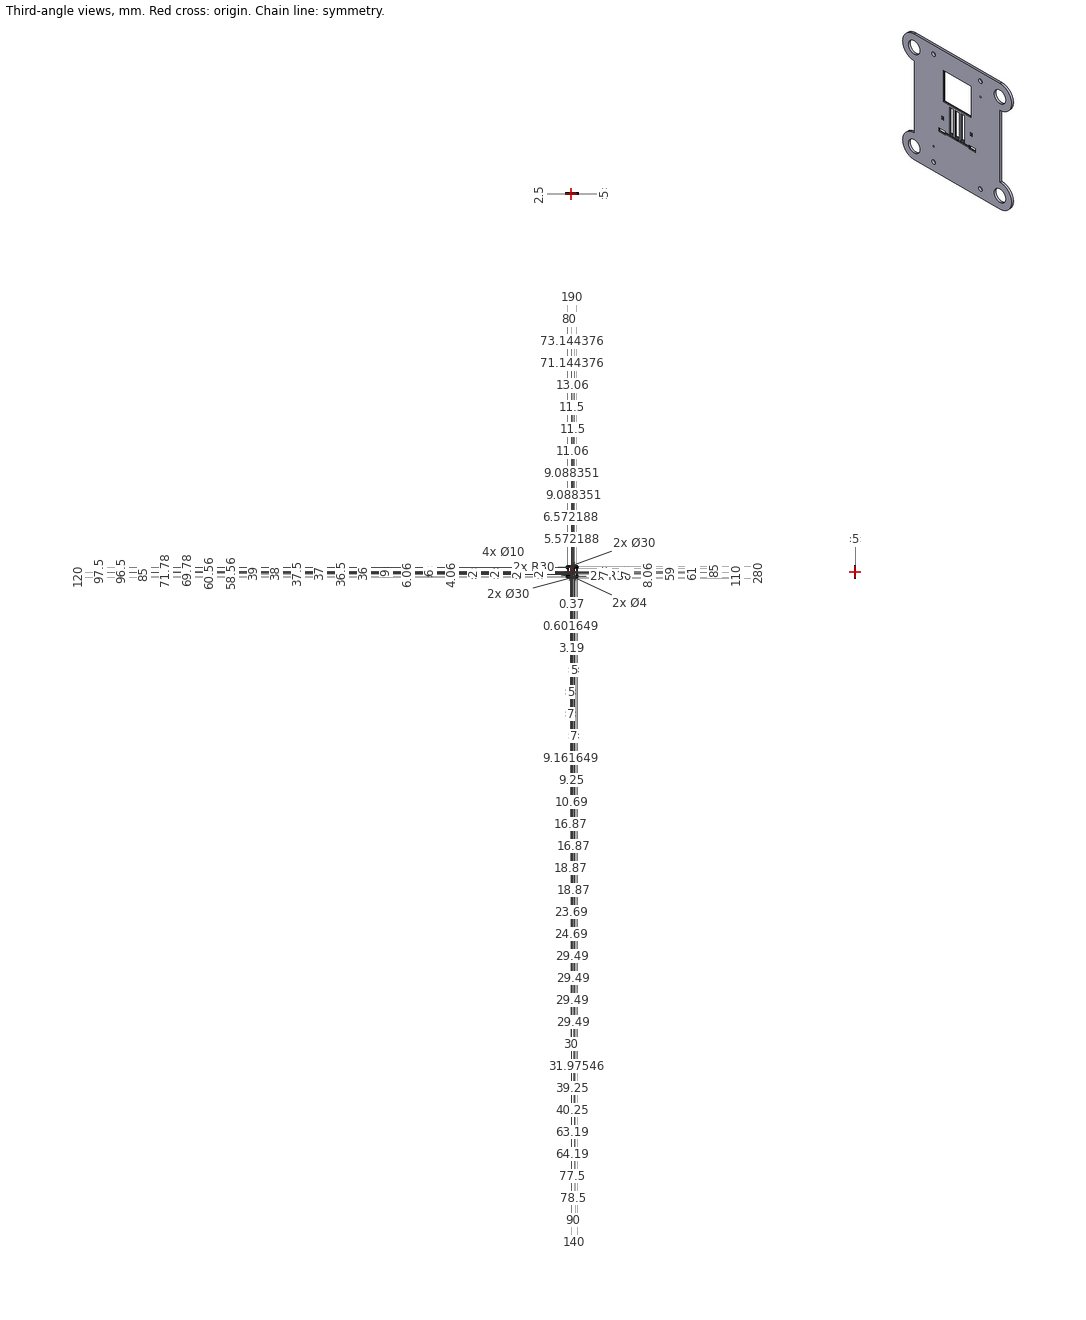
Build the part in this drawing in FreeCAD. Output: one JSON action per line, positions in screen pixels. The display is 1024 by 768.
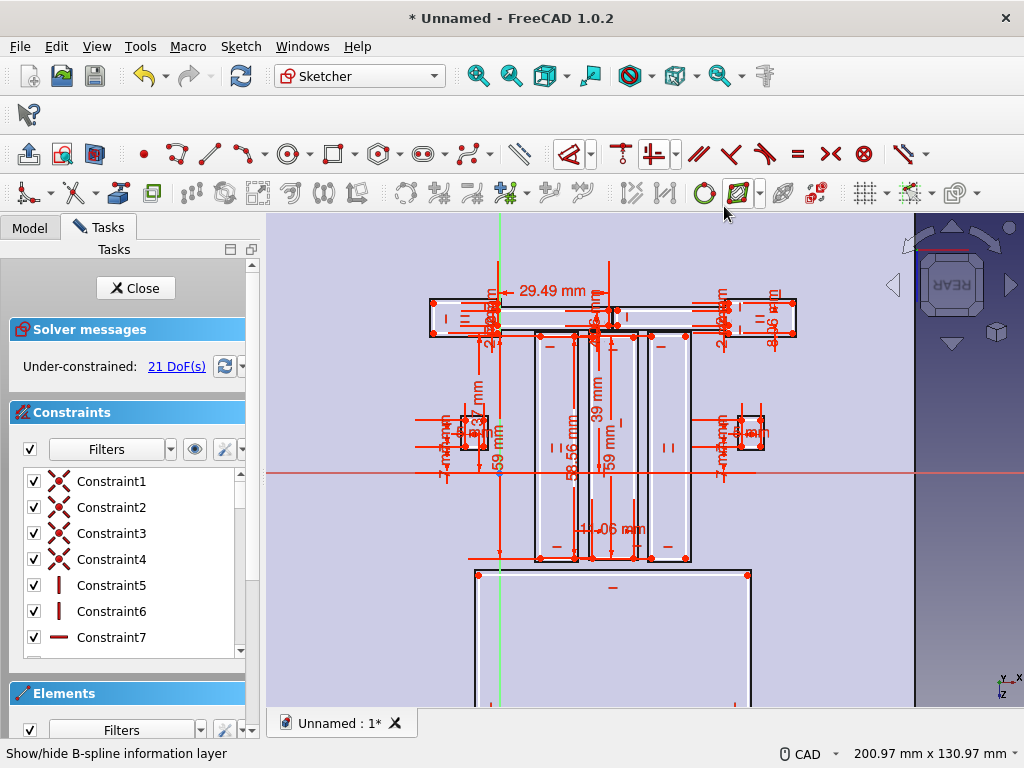
{"action": "left_click", "coordinate": [575, 311]}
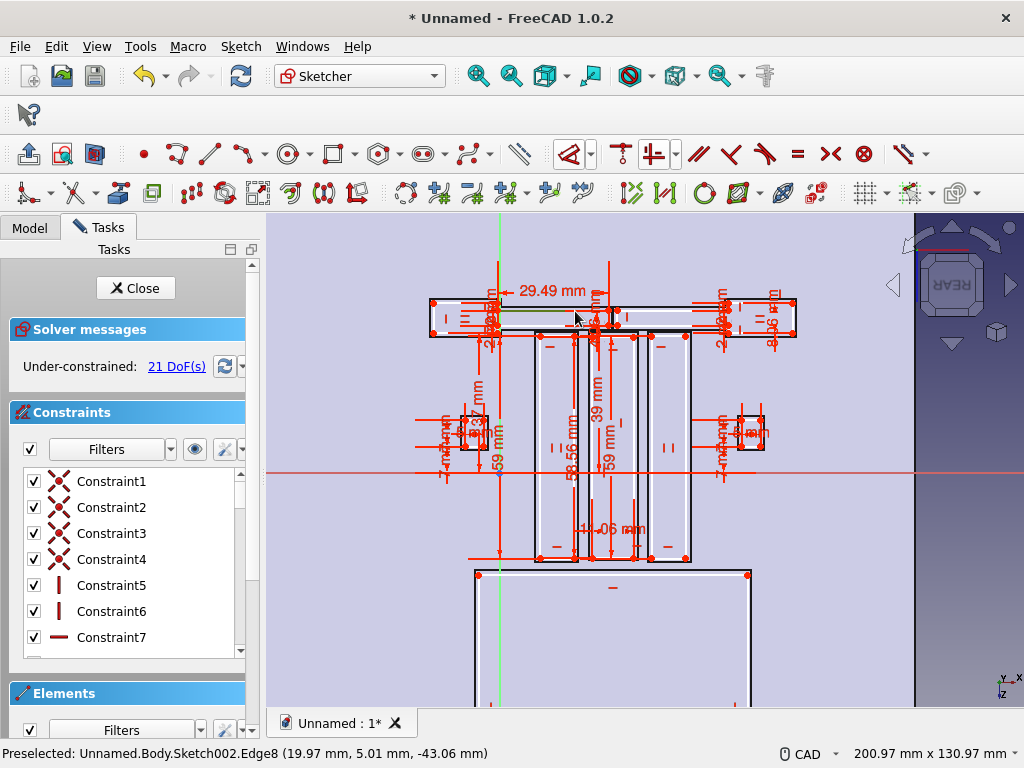
{"action": "left_click", "coordinate": [590, 154]}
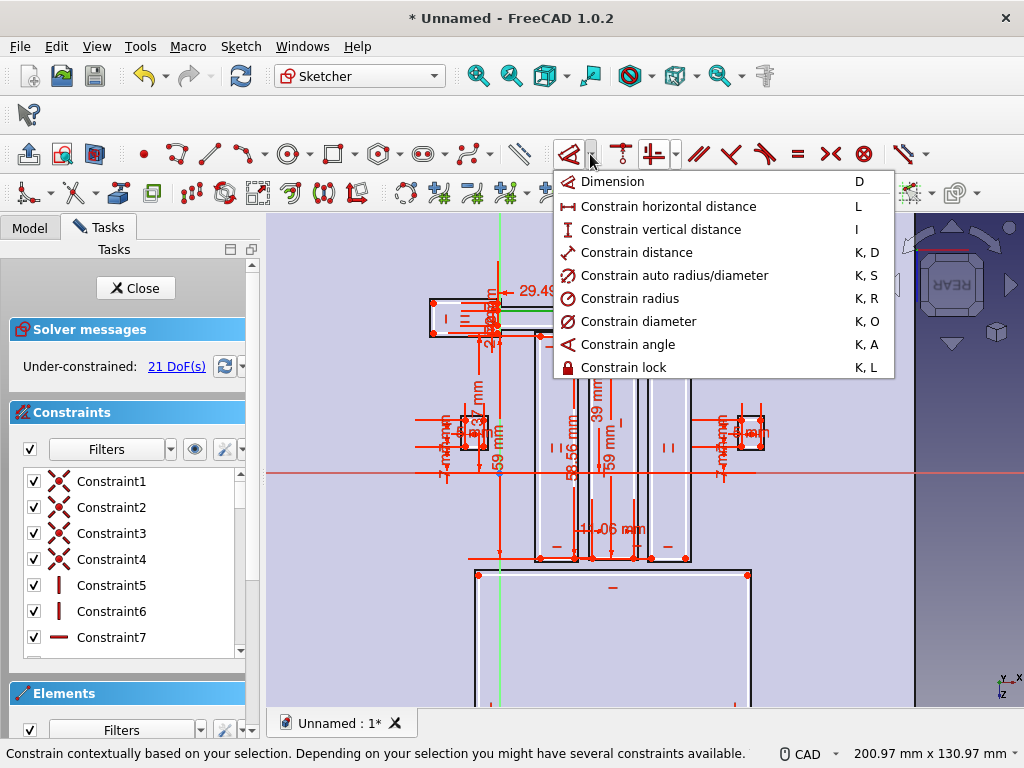
{"action": "left_click", "coordinate": [724, 206]}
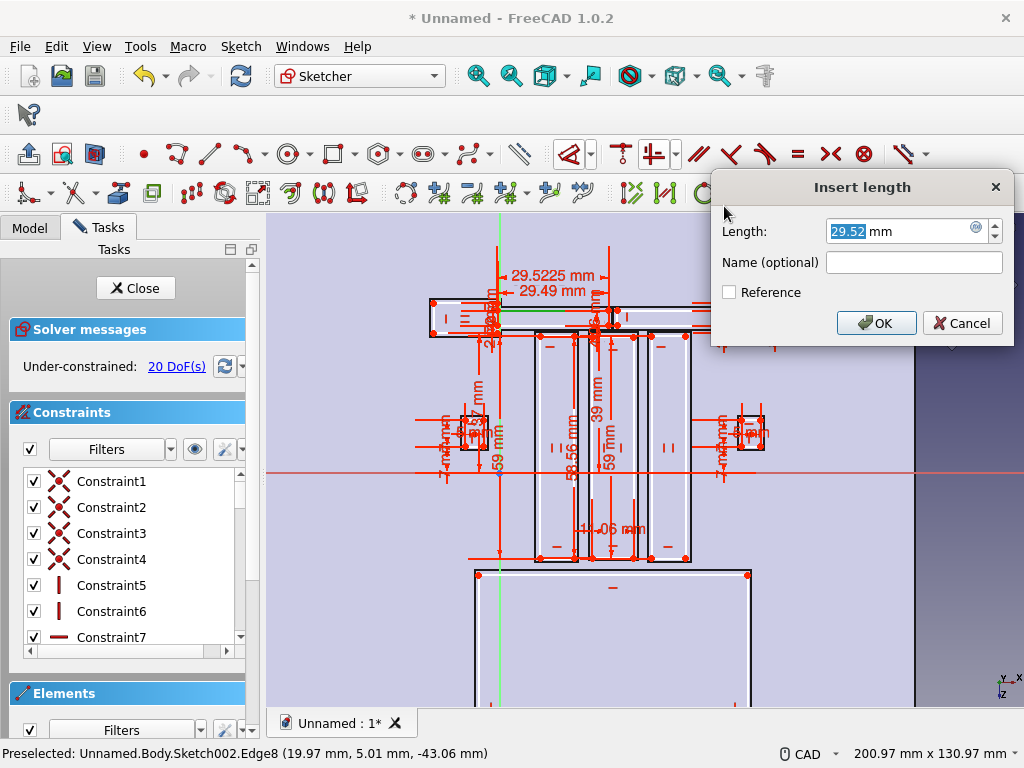
{"action": "type", "text": "29.49"}
{"action": "key", "text": "Return"}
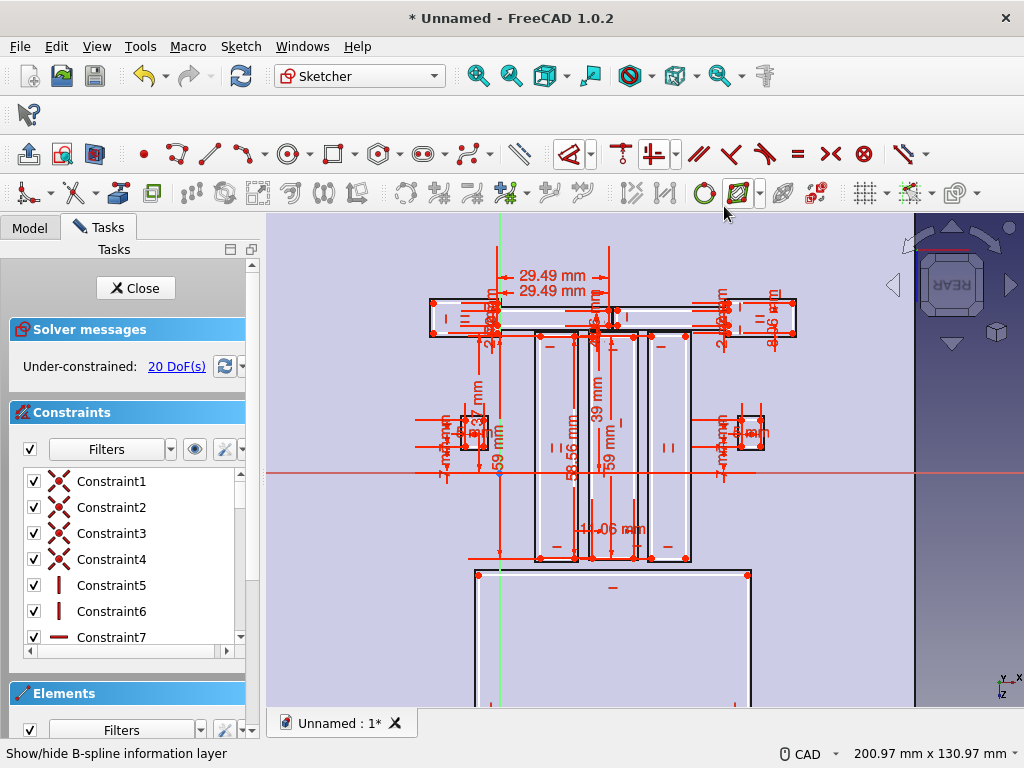
{"action": "left_click", "coordinate": [478, 303]}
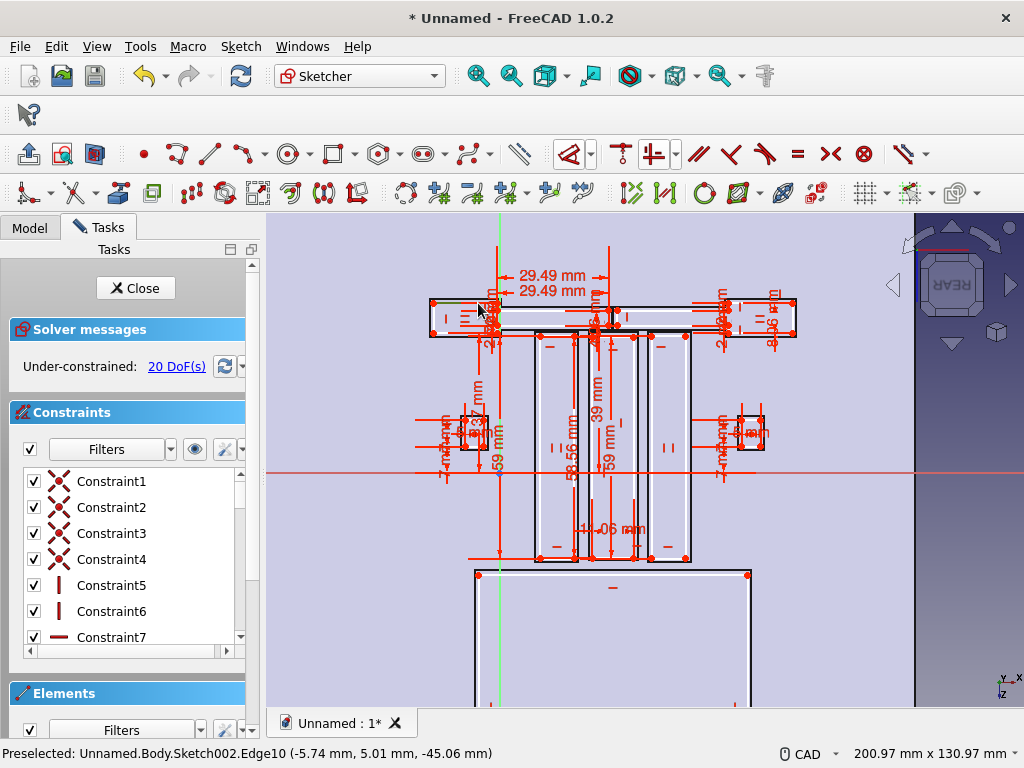
{"action": "left_click", "coordinate": [590, 154]}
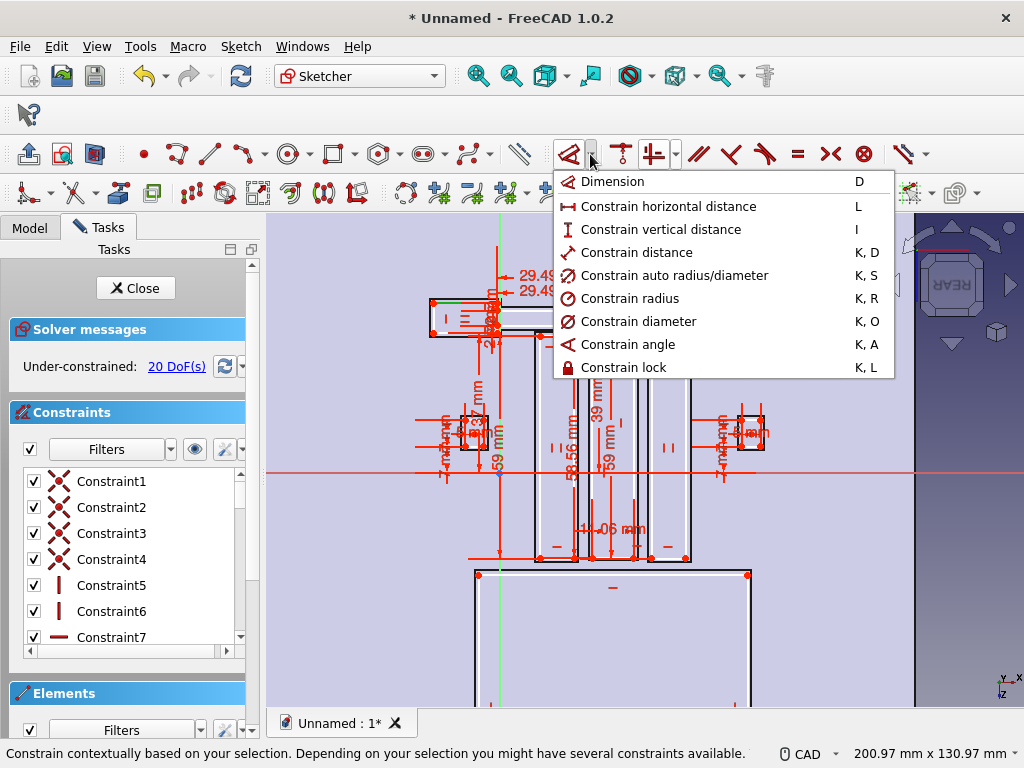
{"action": "left_click", "coordinate": [724, 206]}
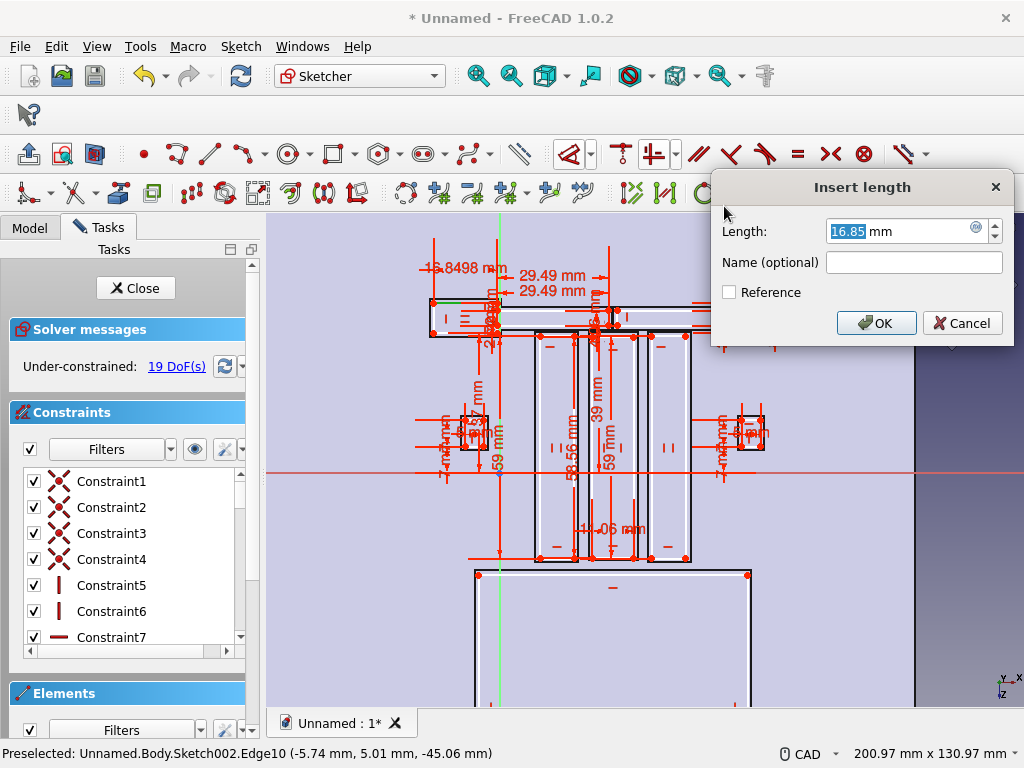
{"action": "type", "text": "16.87"}
{"action": "key", "text": "Return"}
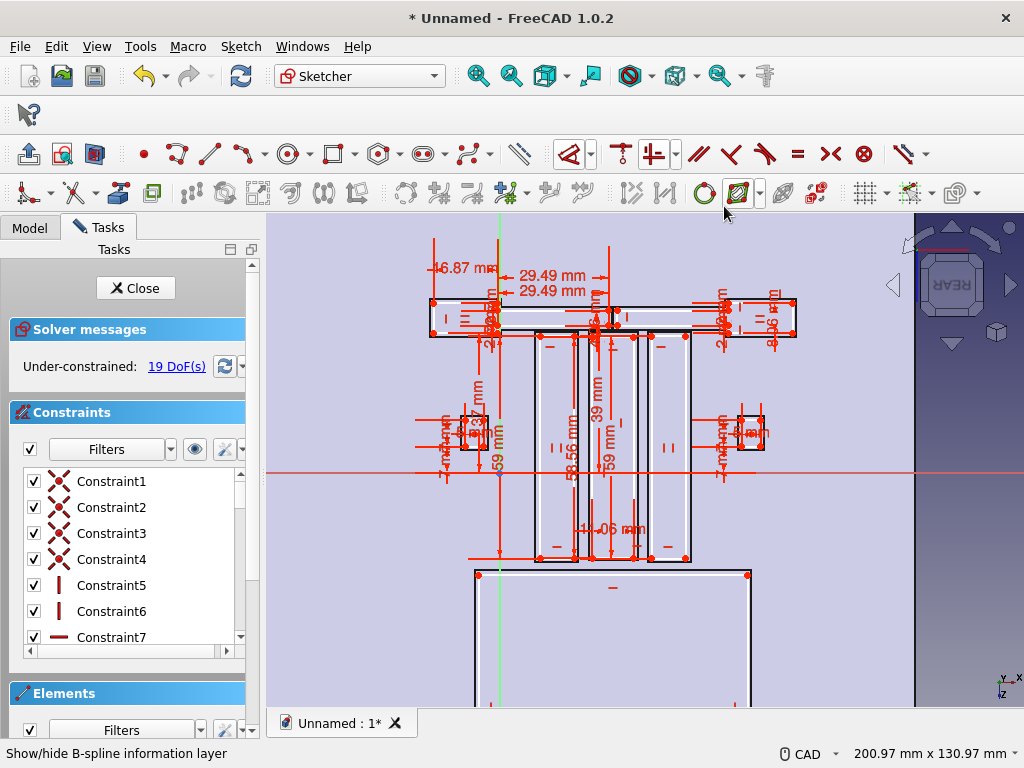
{"action": "scroll", "coordinate": [651, 326], "scroll_direction": "up", "scroll_amount": 2}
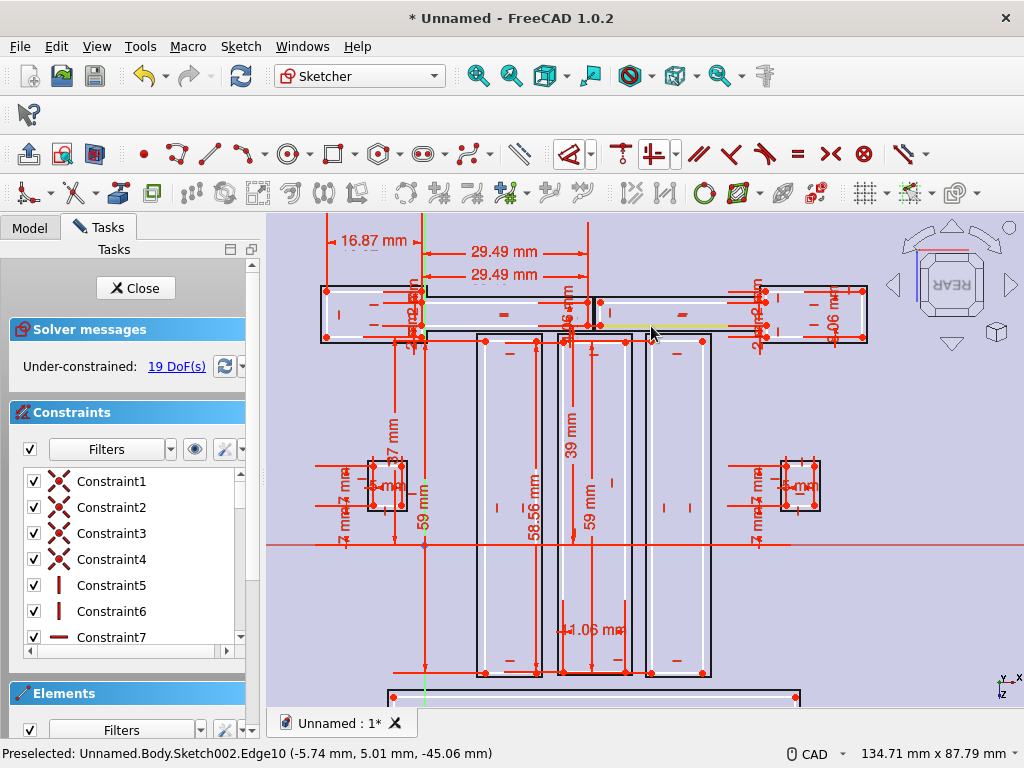
{"action": "left_click", "coordinate": [650, 326]}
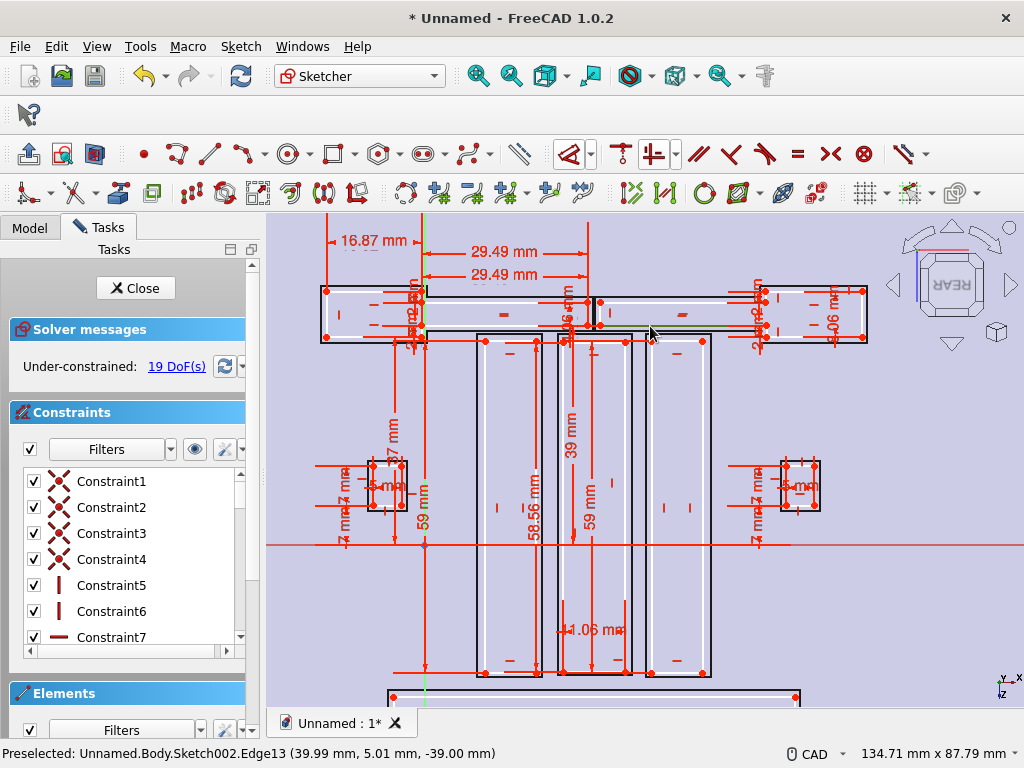
{"action": "key", "text": "l"}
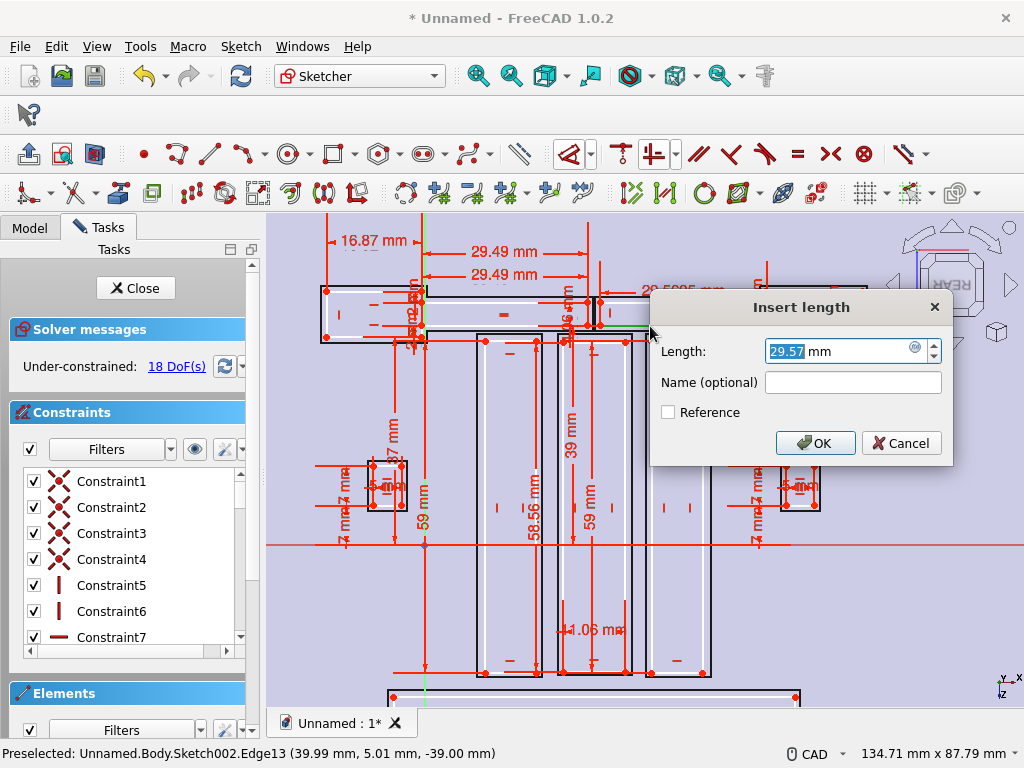
{"action": "type", "text": "29.49"}
{"action": "key", "text": "Return"}